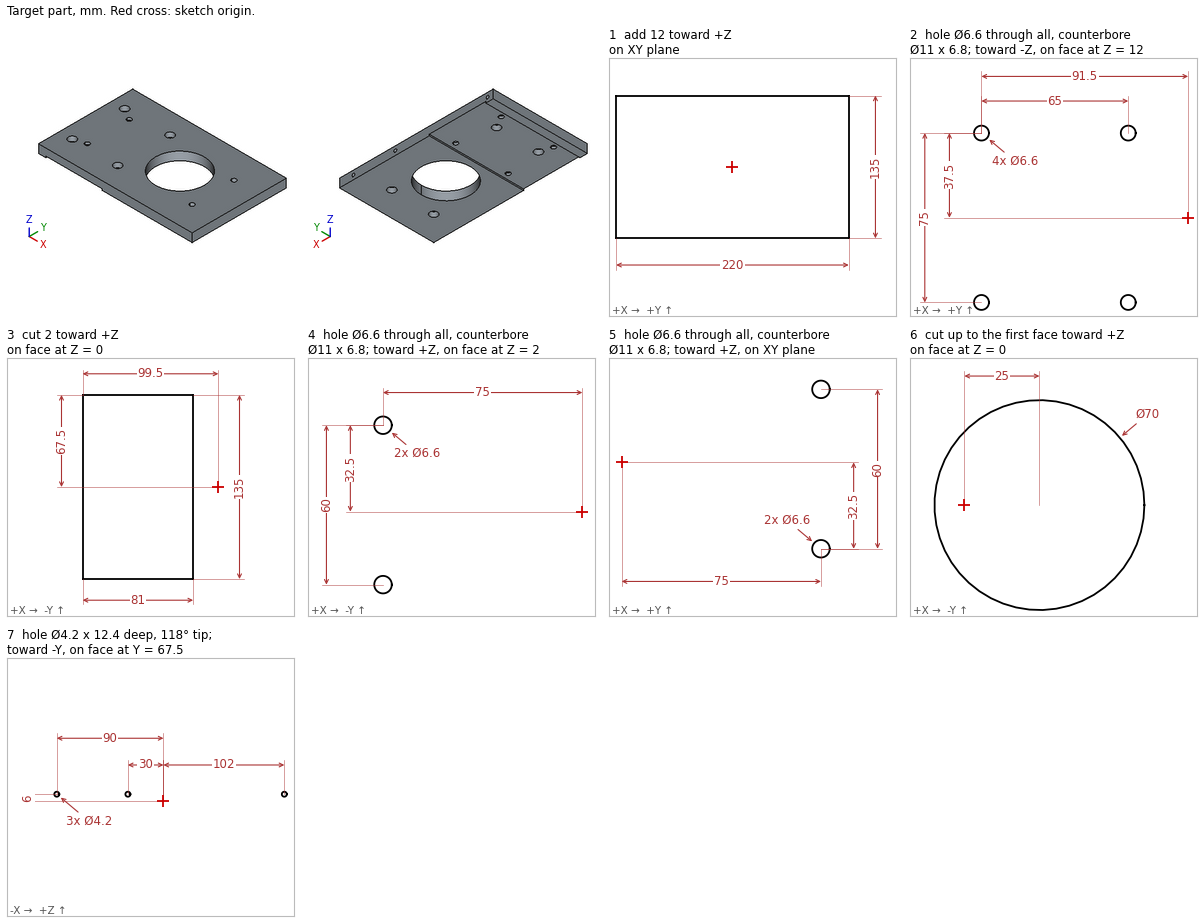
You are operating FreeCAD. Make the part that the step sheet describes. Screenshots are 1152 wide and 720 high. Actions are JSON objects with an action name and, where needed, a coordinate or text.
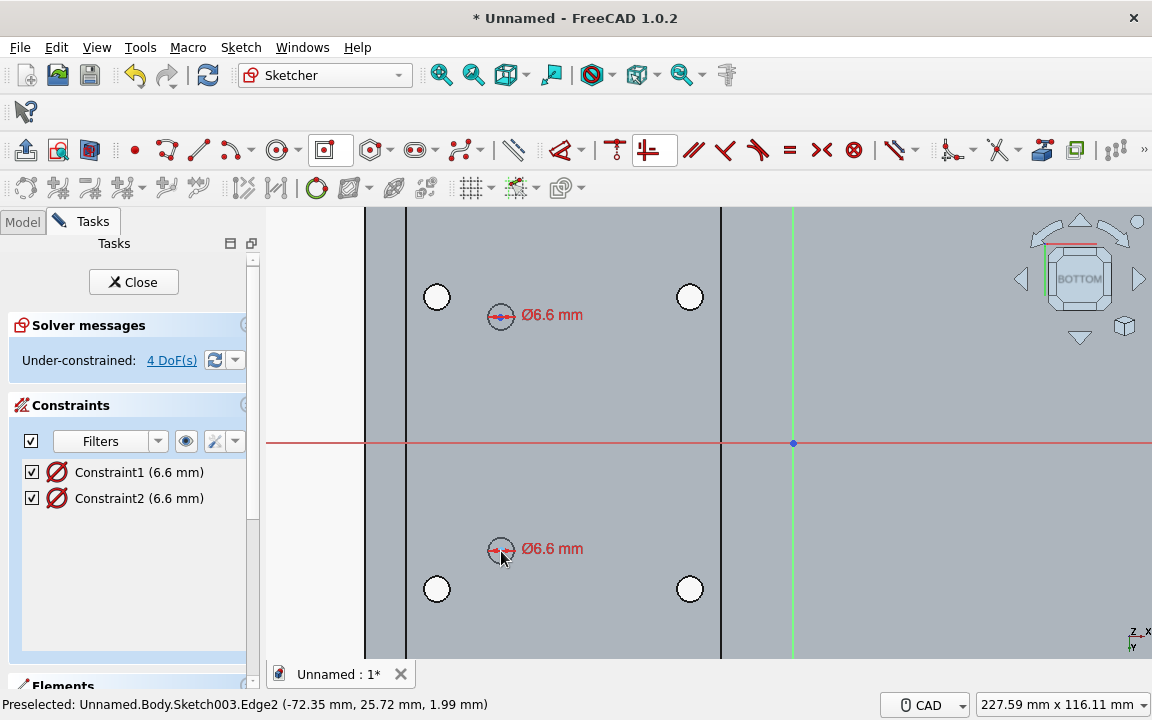
{"action": "left_click", "coordinate": [501, 317]}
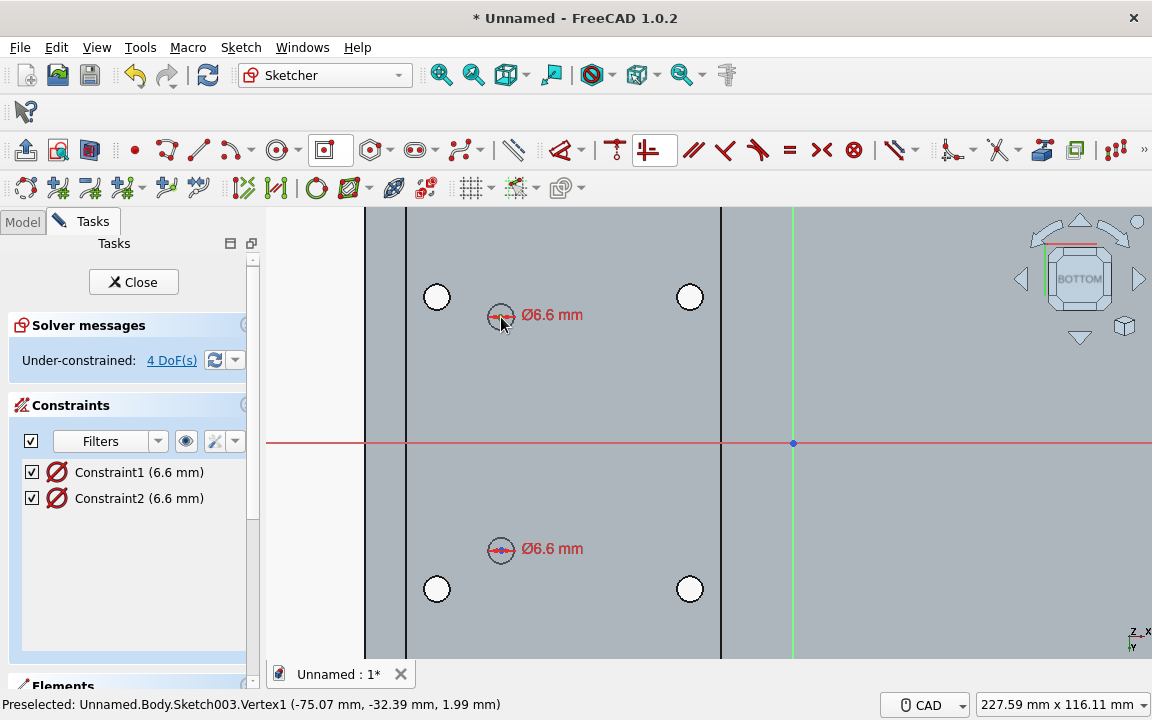
{"action": "left_click", "coordinate": [501, 551]}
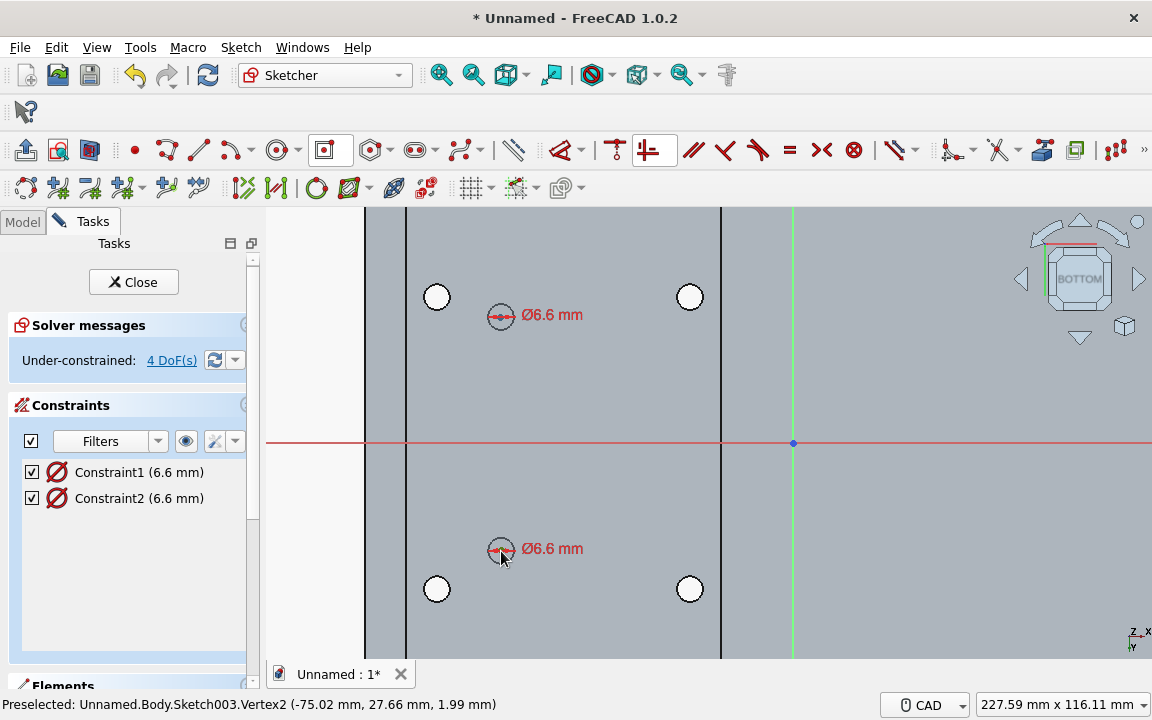
{"action": "key", "text": "v"}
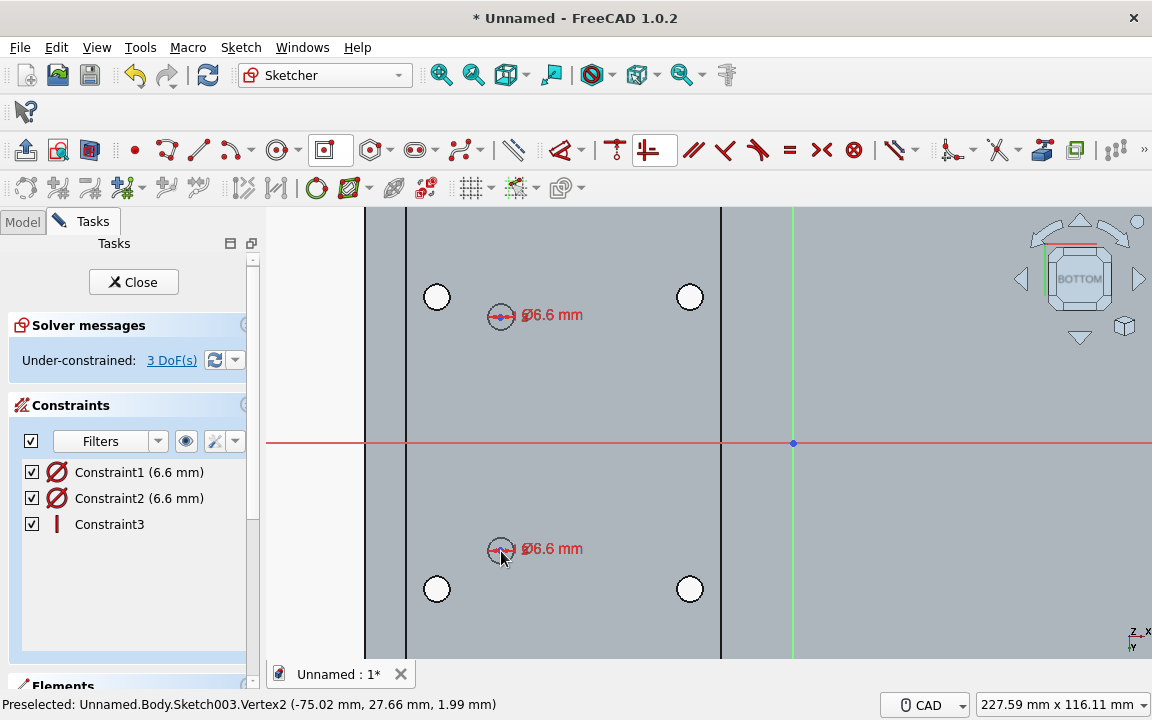
{"action": "key", "text": "d"}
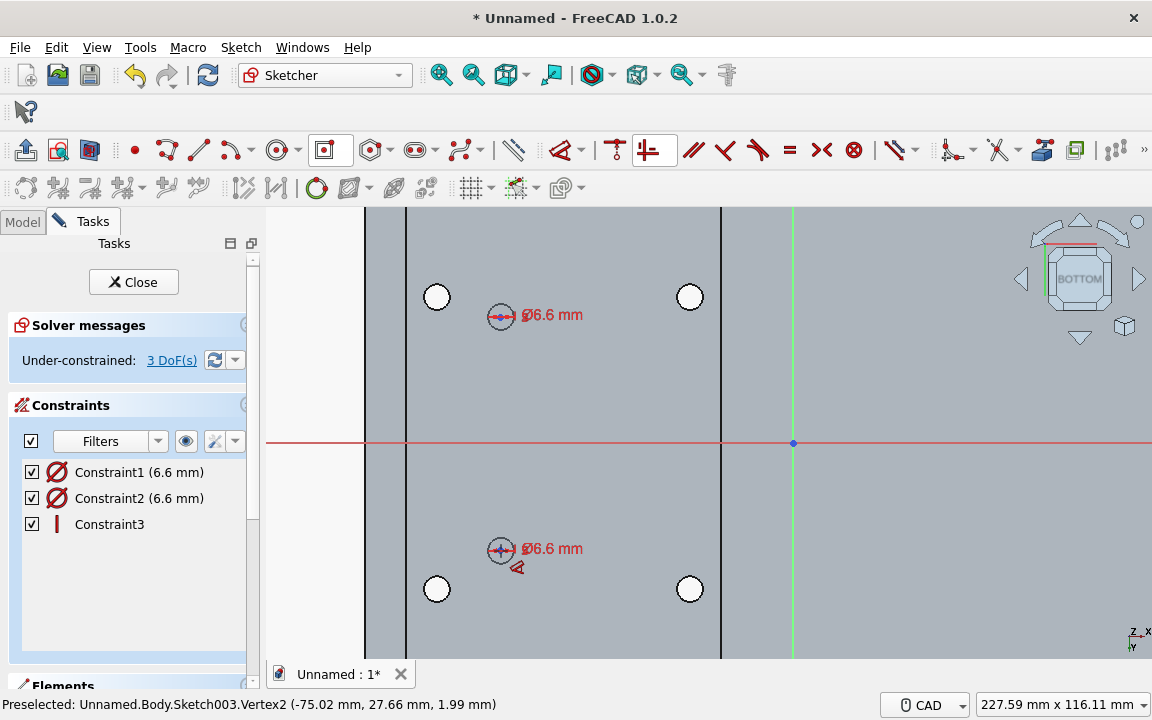
{"action": "left_click", "coordinate": [501, 317]}
{"action": "left_click", "coordinate": [647, 283]}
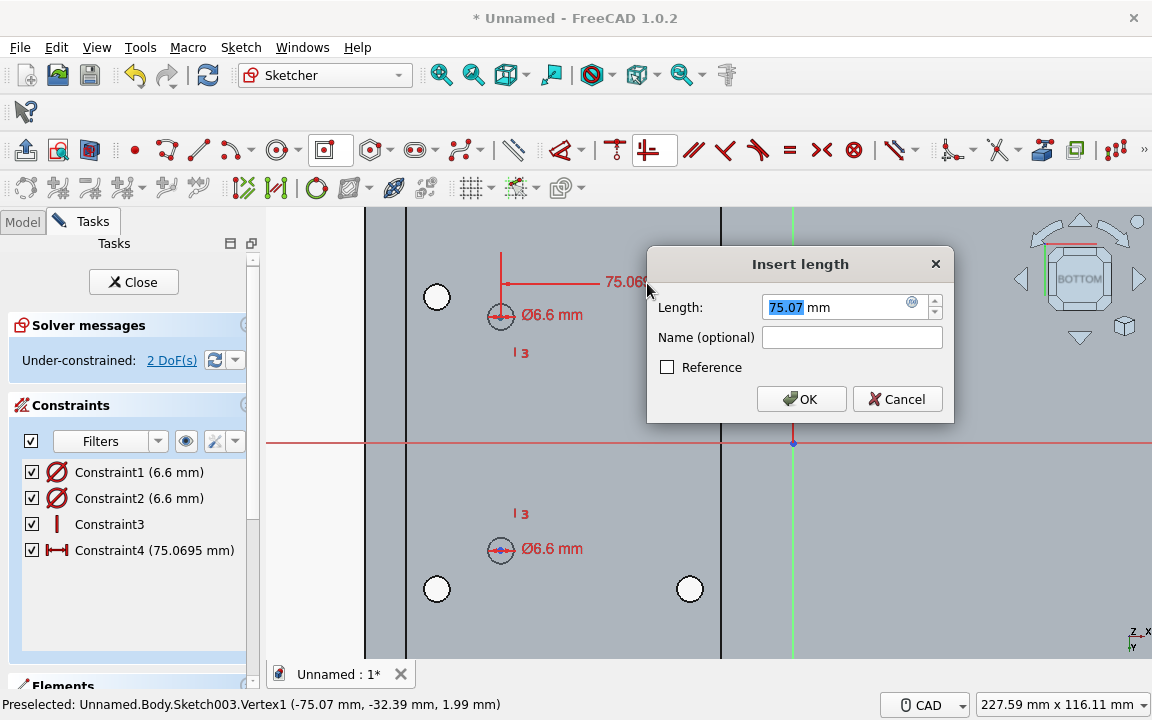
{"action": "type", "text": "75"}
{"action": "key", "text": "Return"}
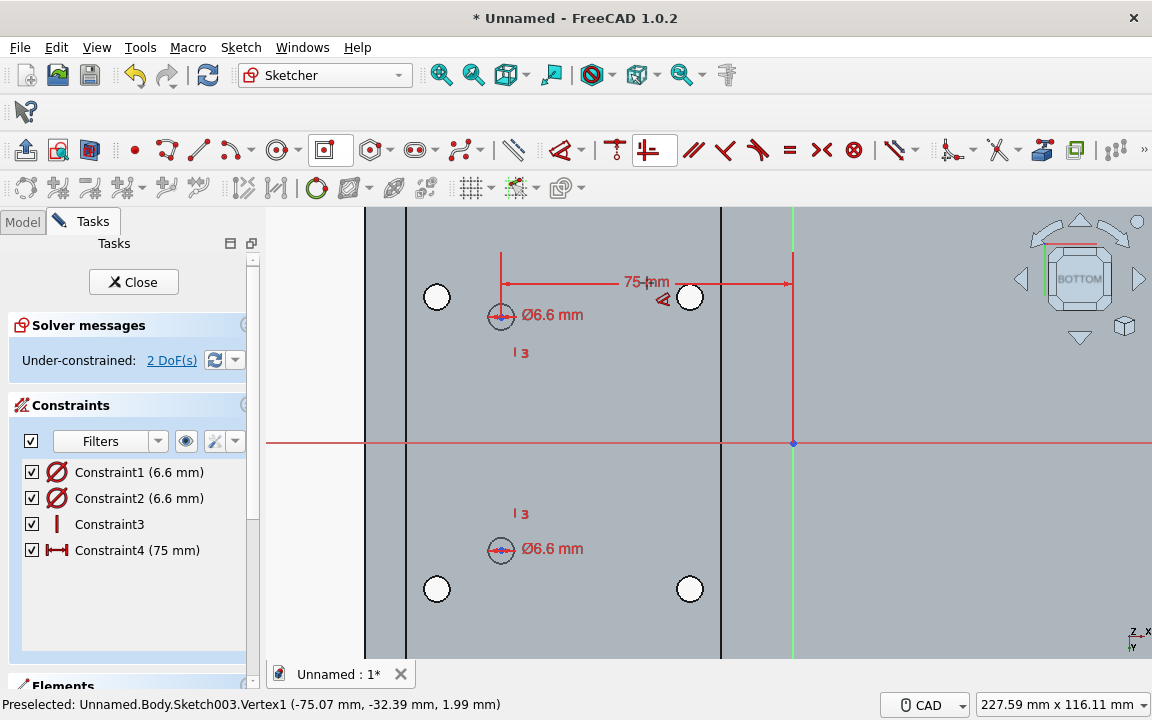
{"action": "left_click", "coordinate": [501, 317]}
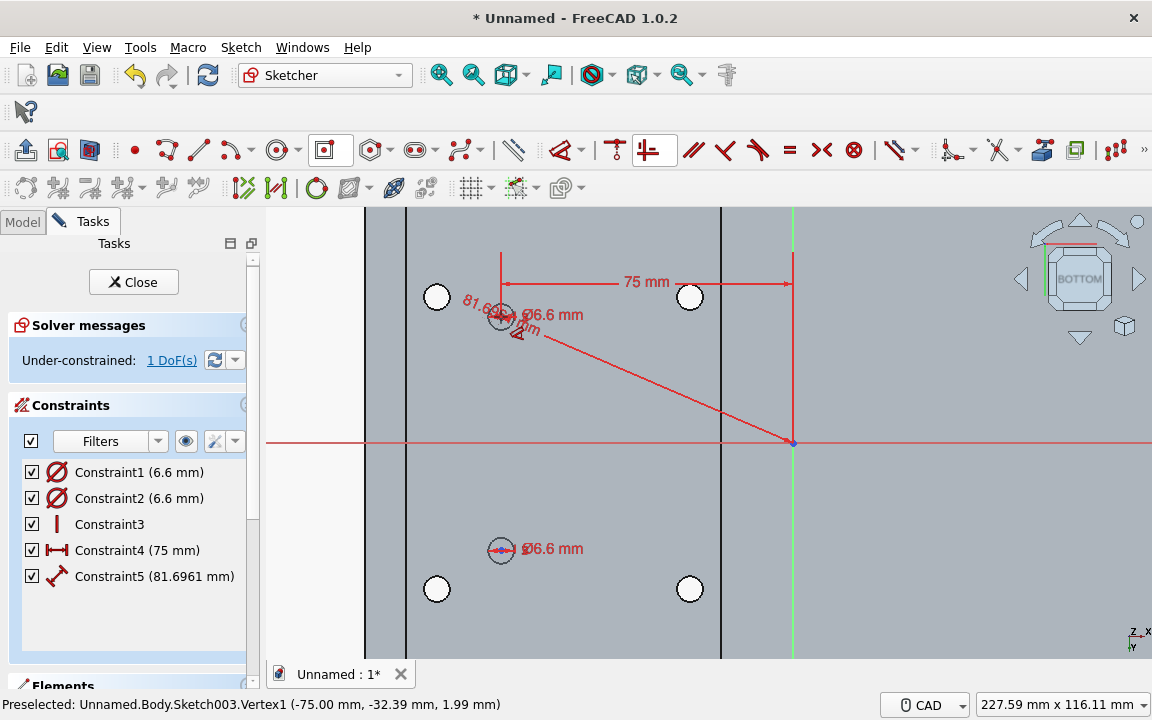
{"action": "left_click", "coordinate": [501, 551]}
{"action": "left_click", "coordinate": [467, 380]}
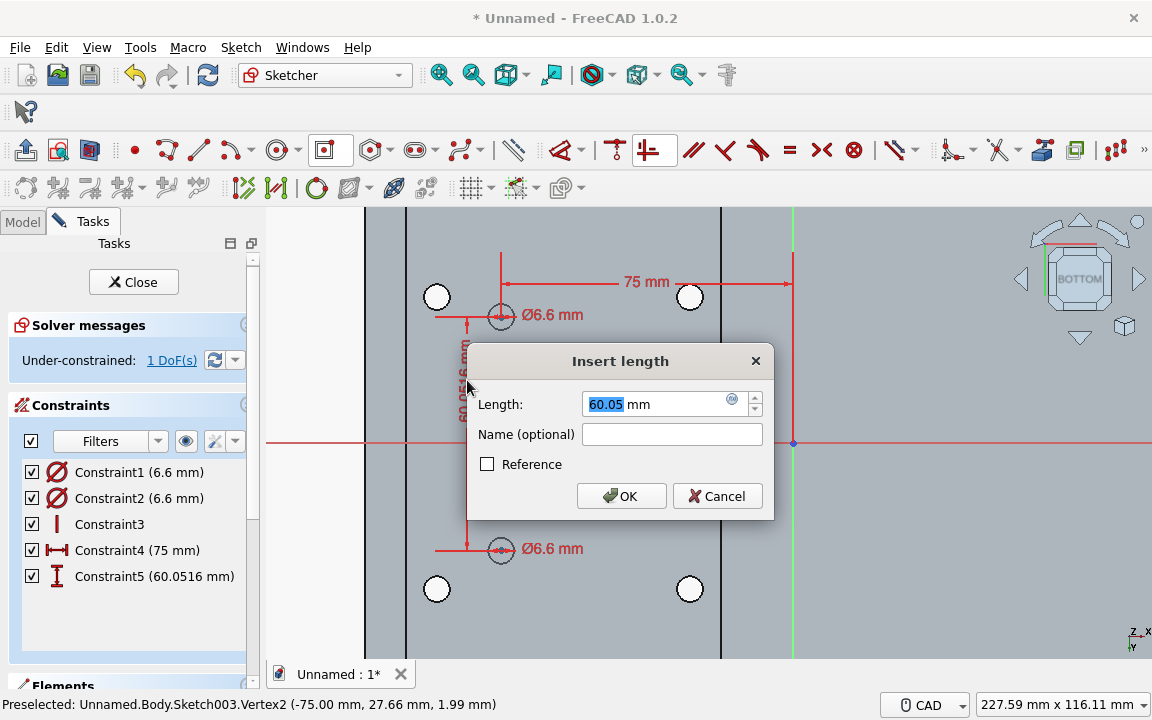
{"action": "type", "text": "60"}
{"action": "key", "text": "Return"}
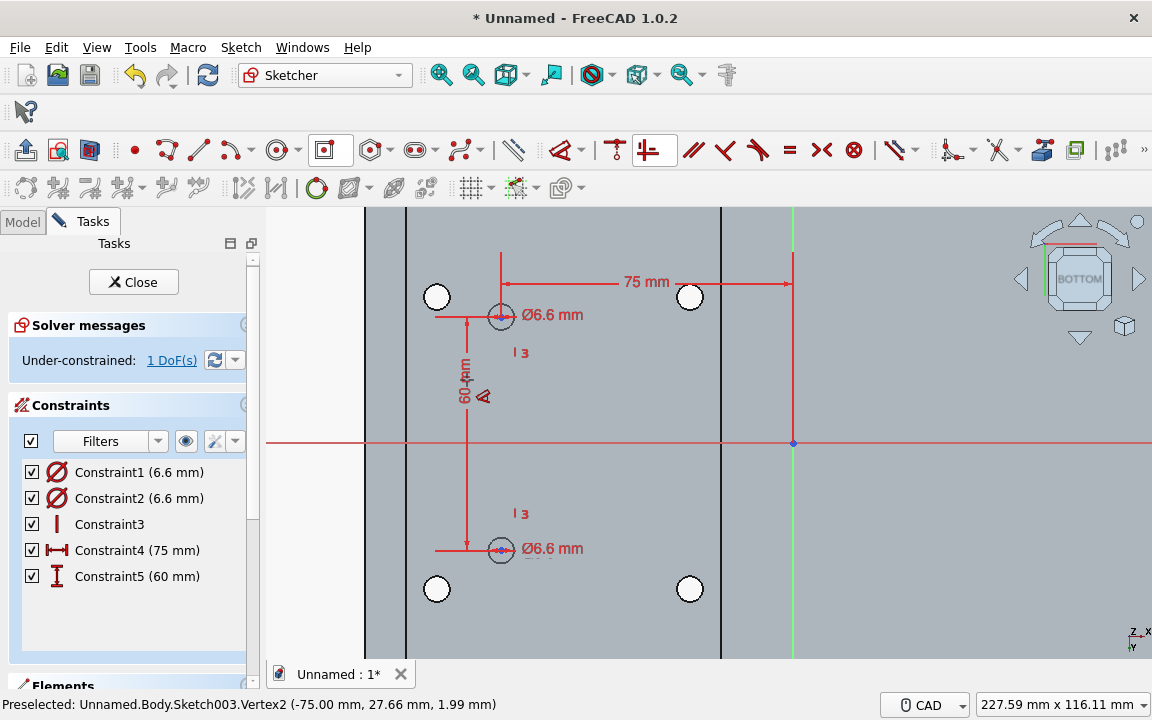
{"action": "left_click", "coordinate": [501, 317]}
{"action": "left_click", "coordinate": [827, 380]}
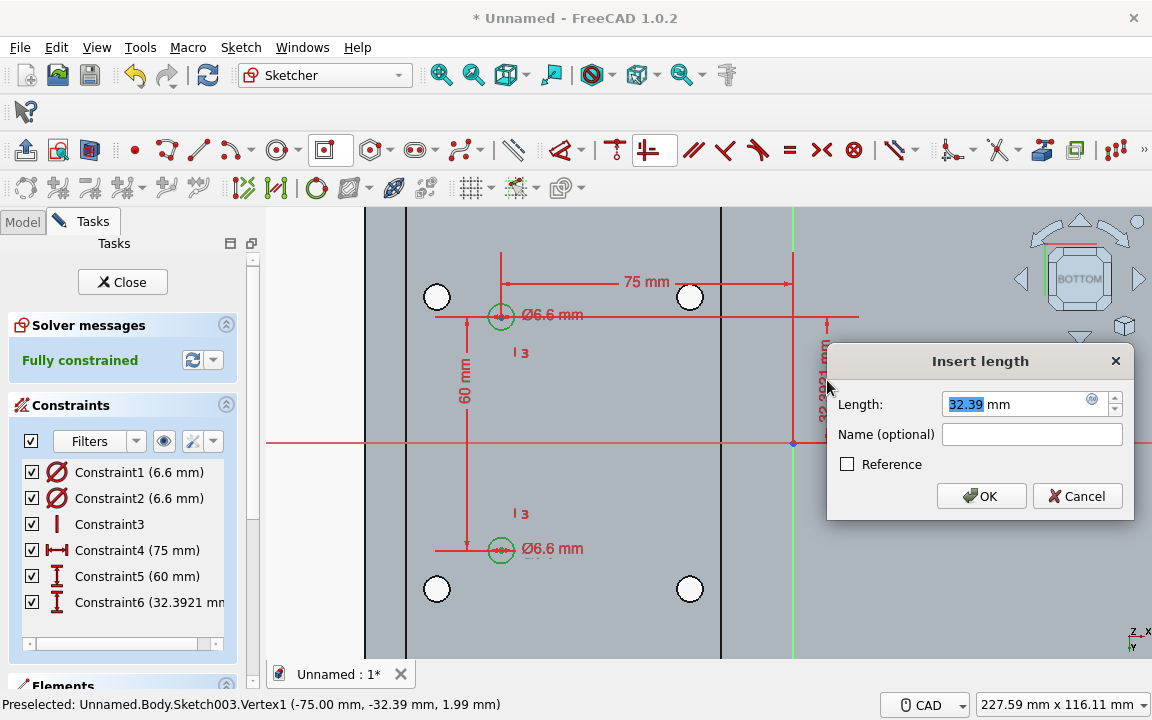
{"action": "type", "text": "32.5"}
{"action": "key", "text": "Return"}
{"action": "key", "text": "Escape"}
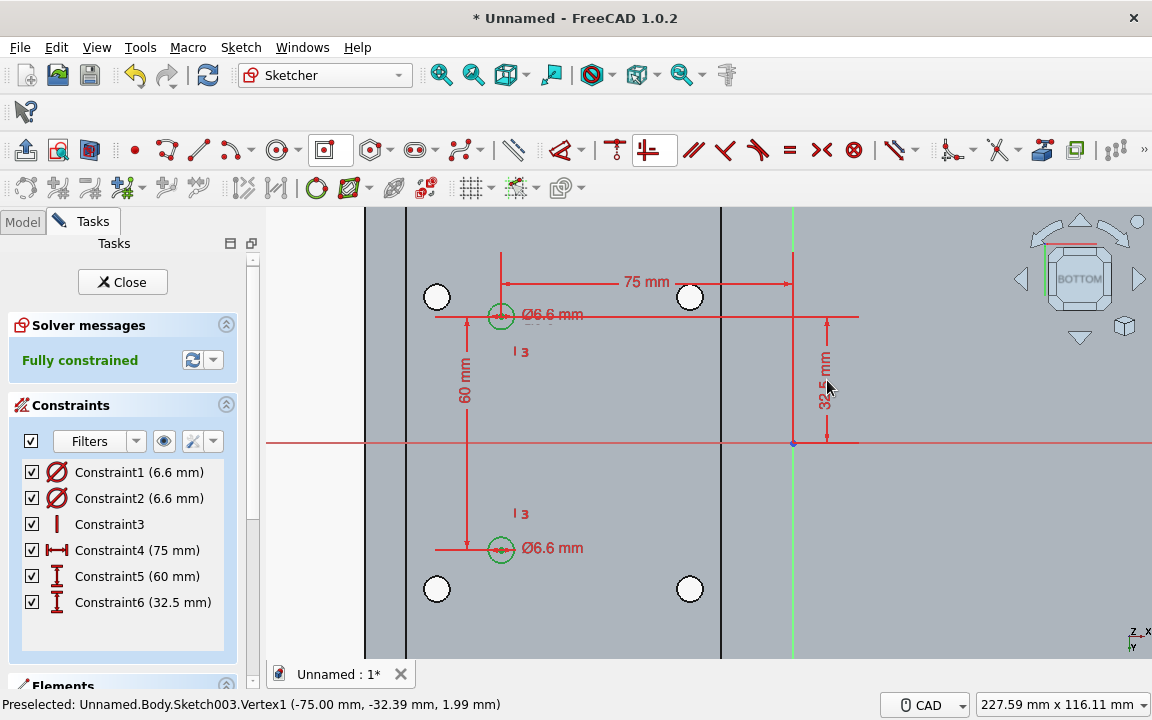
{"action": "left_click", "coordinate": [123, 282]}